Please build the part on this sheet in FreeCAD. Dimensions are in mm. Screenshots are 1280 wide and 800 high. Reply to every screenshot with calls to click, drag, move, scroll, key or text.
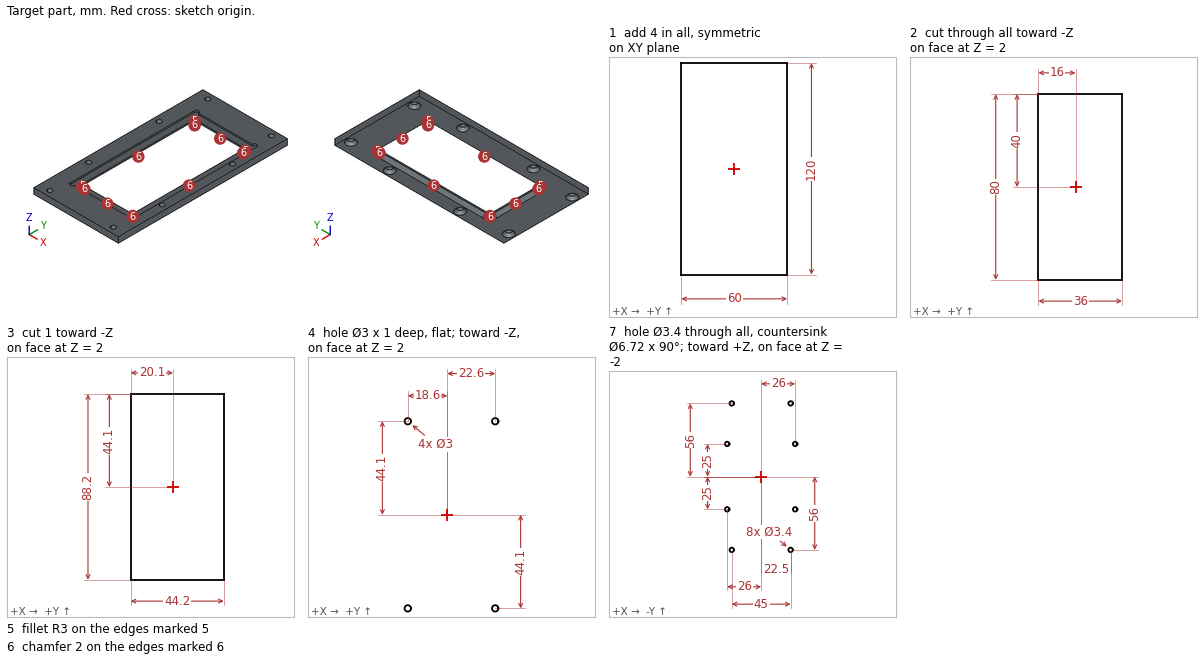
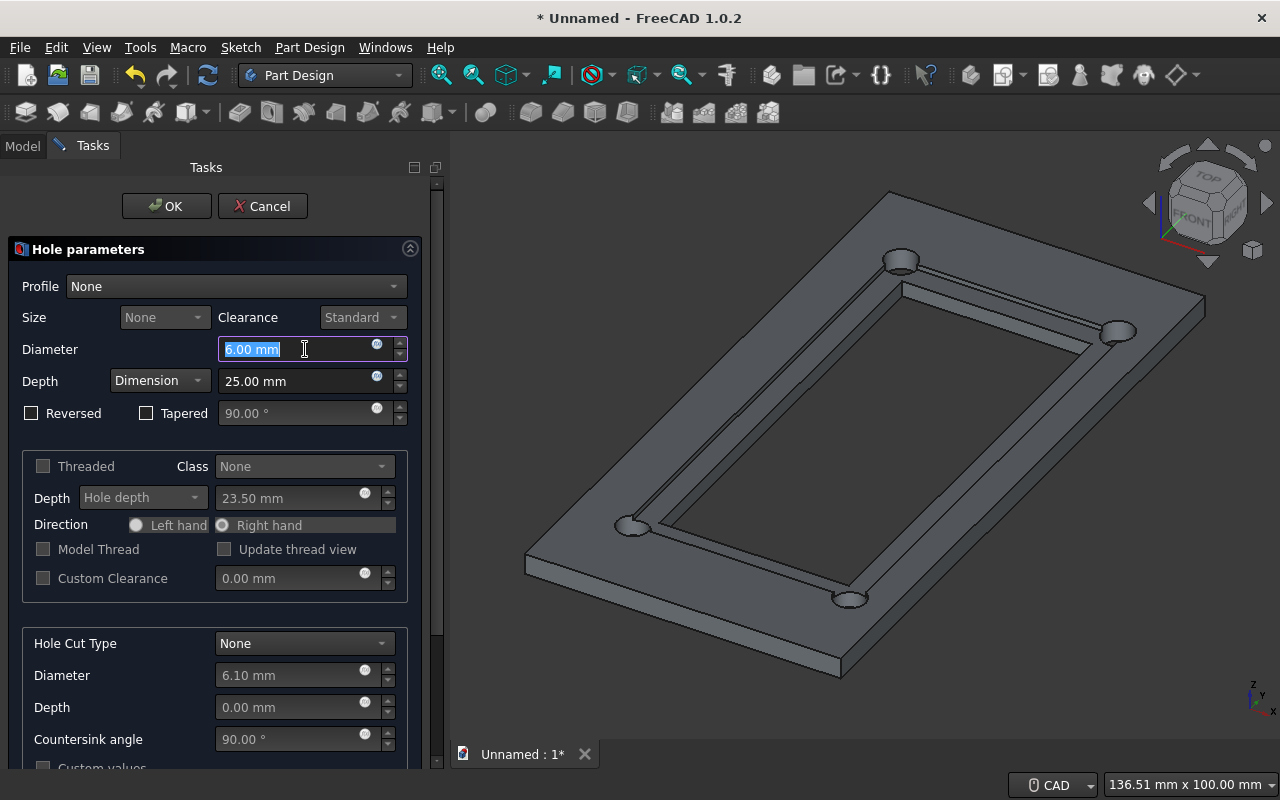
text(3)
key(Tab)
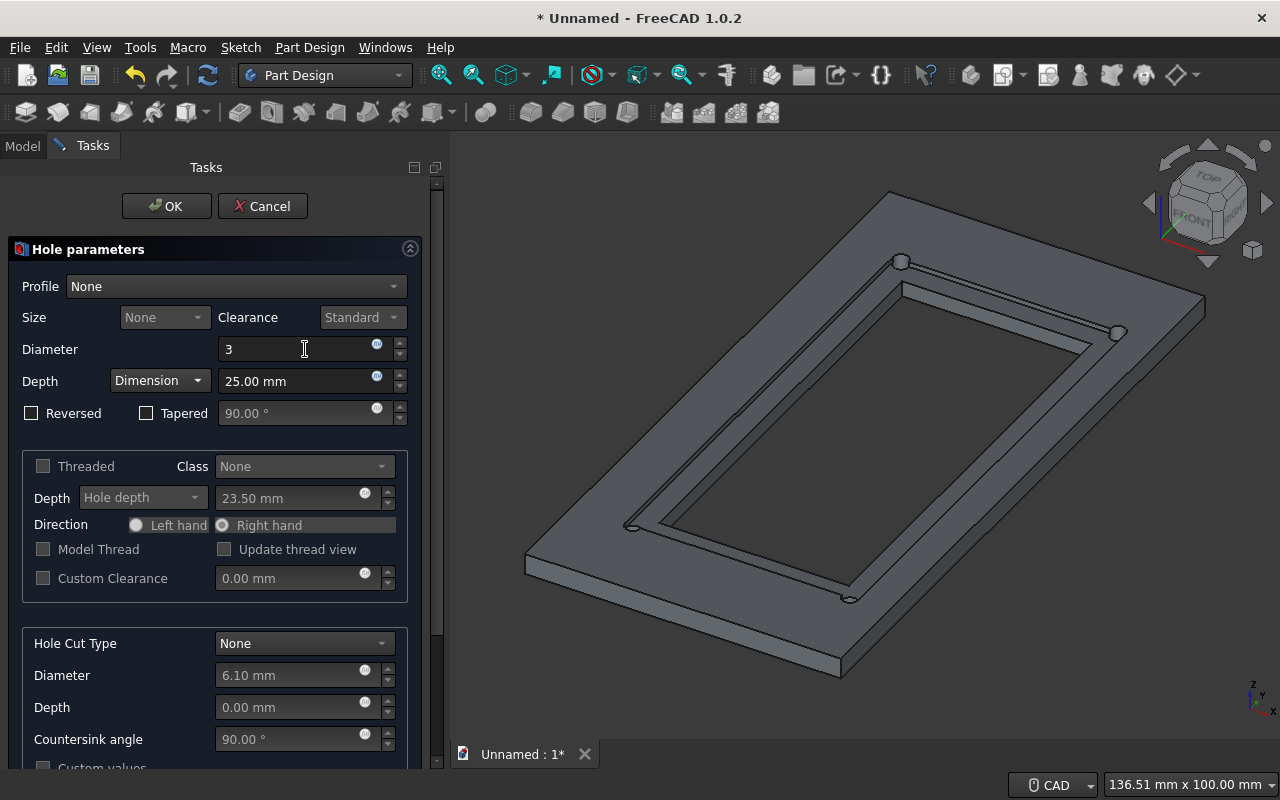
triple_click(305, 381)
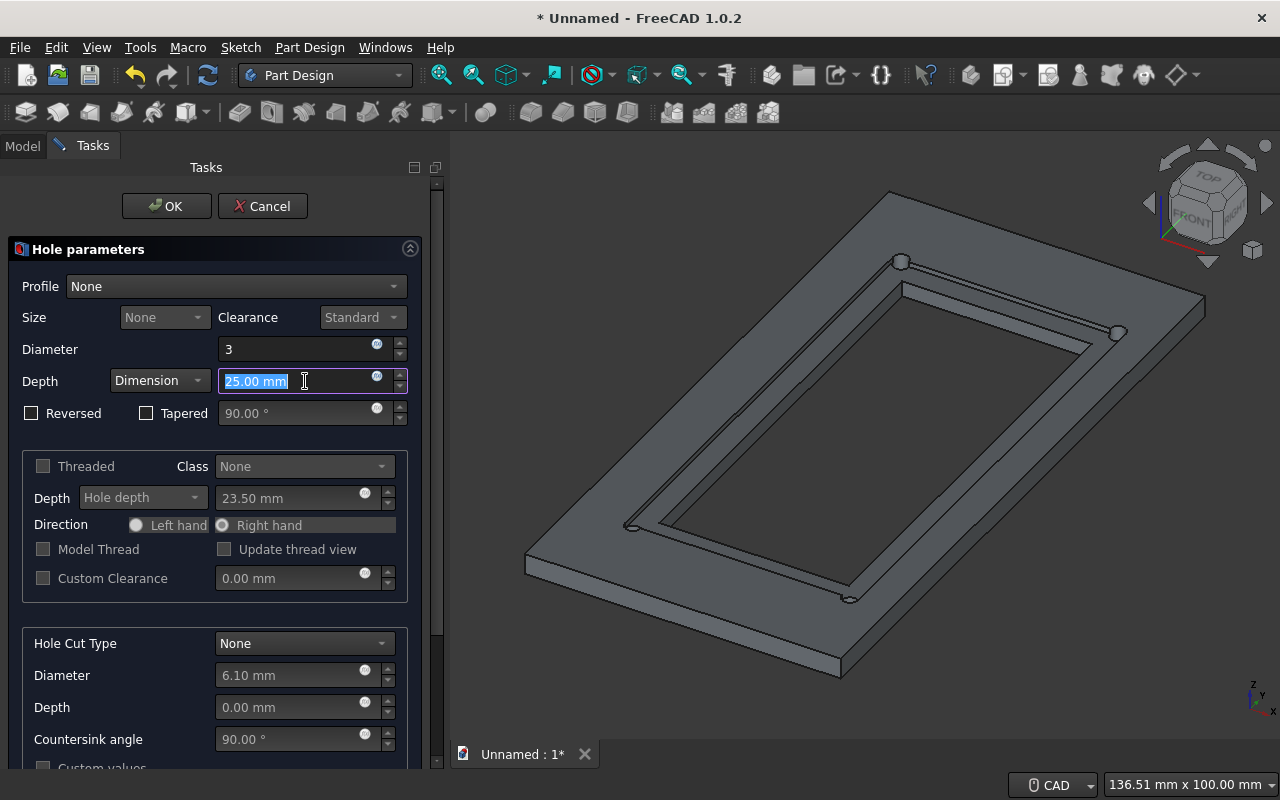
text(1)
key(Tab)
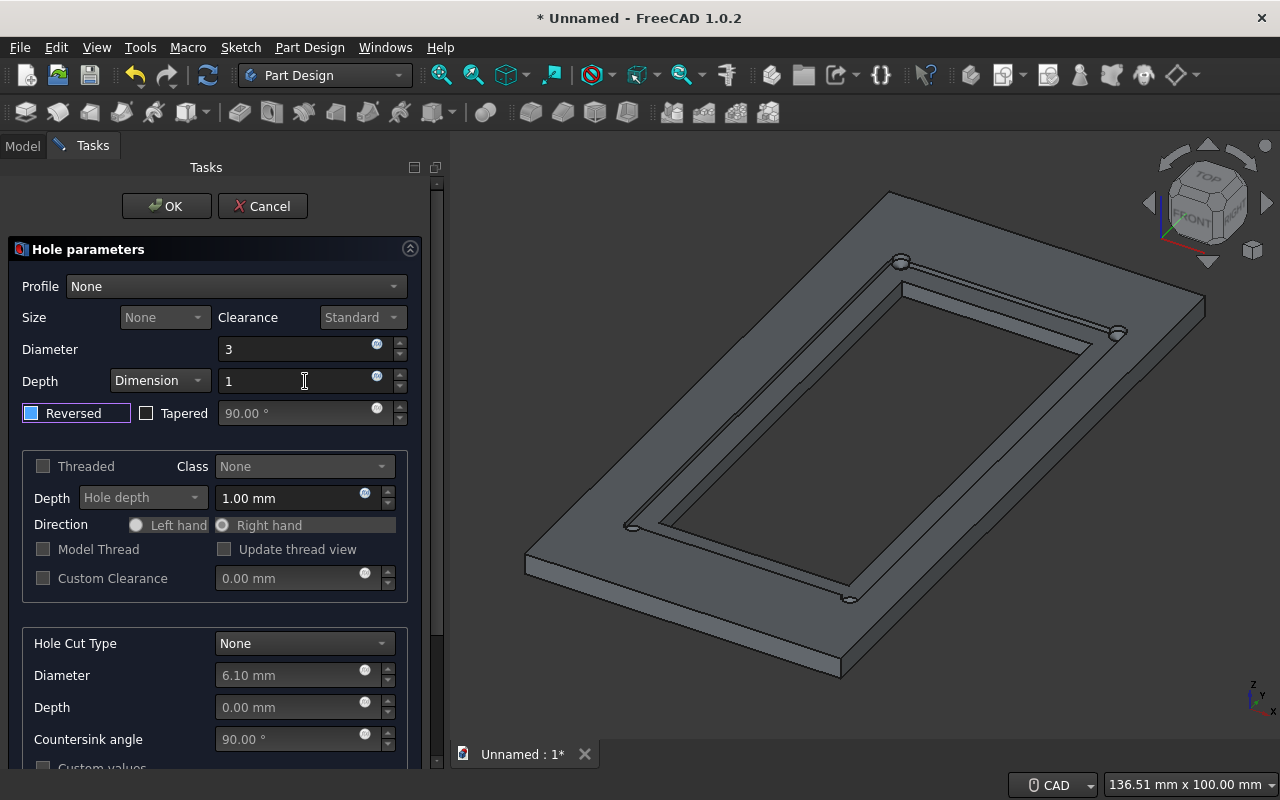
scroll(437, 472, down, 3)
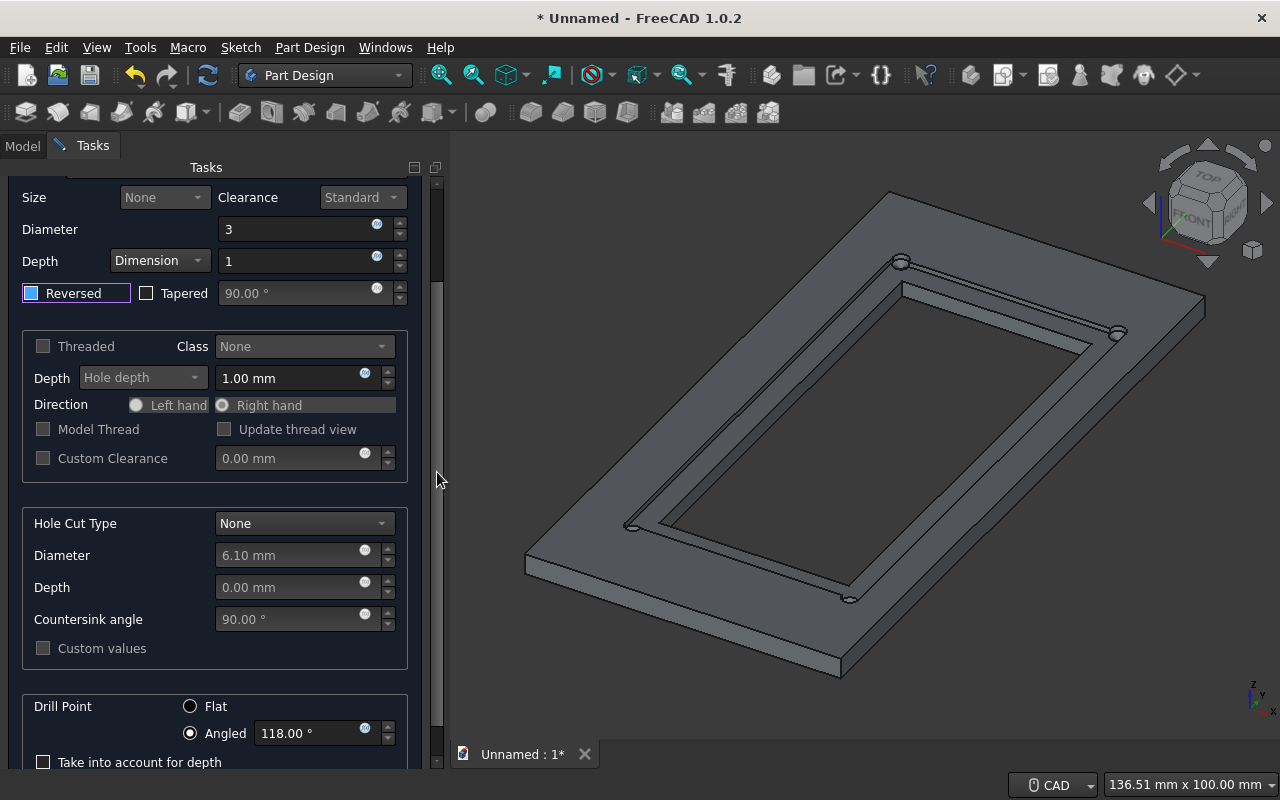
click(191, 669)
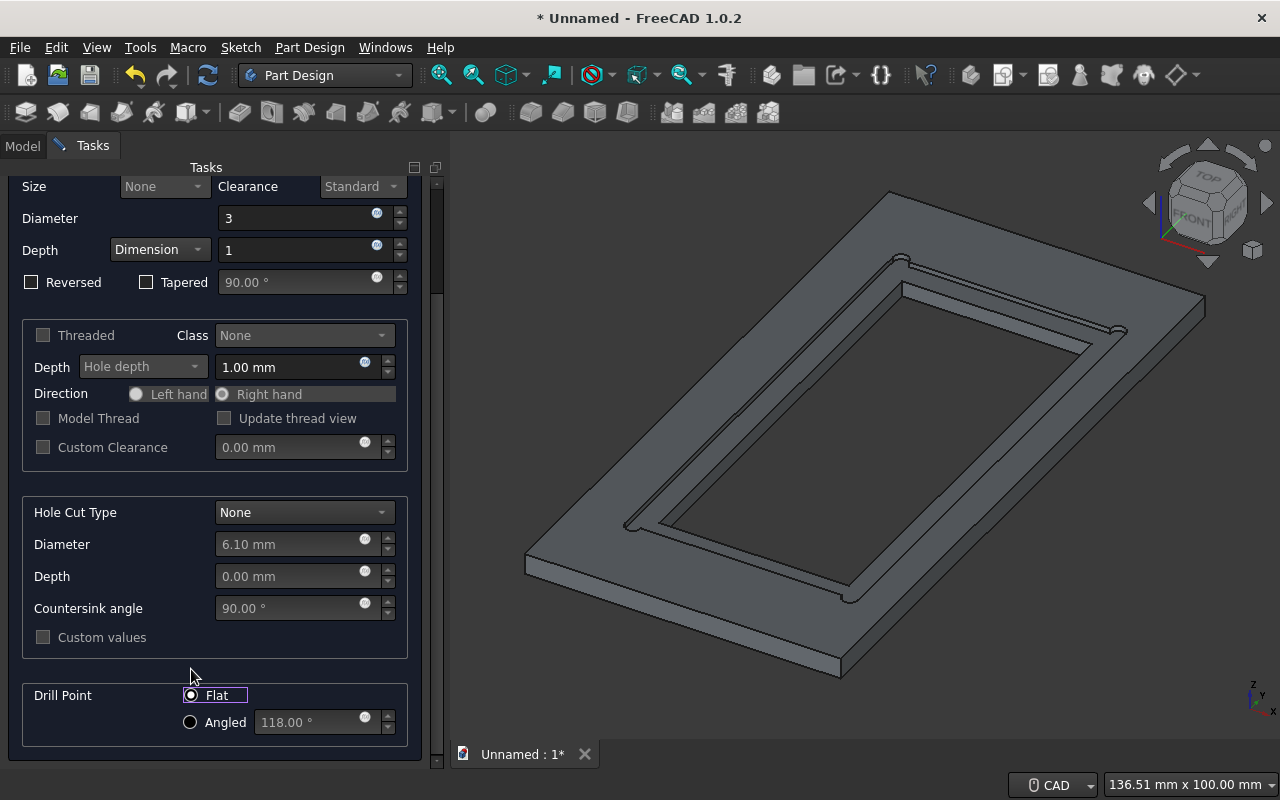
scroll(437, 472, up, 3)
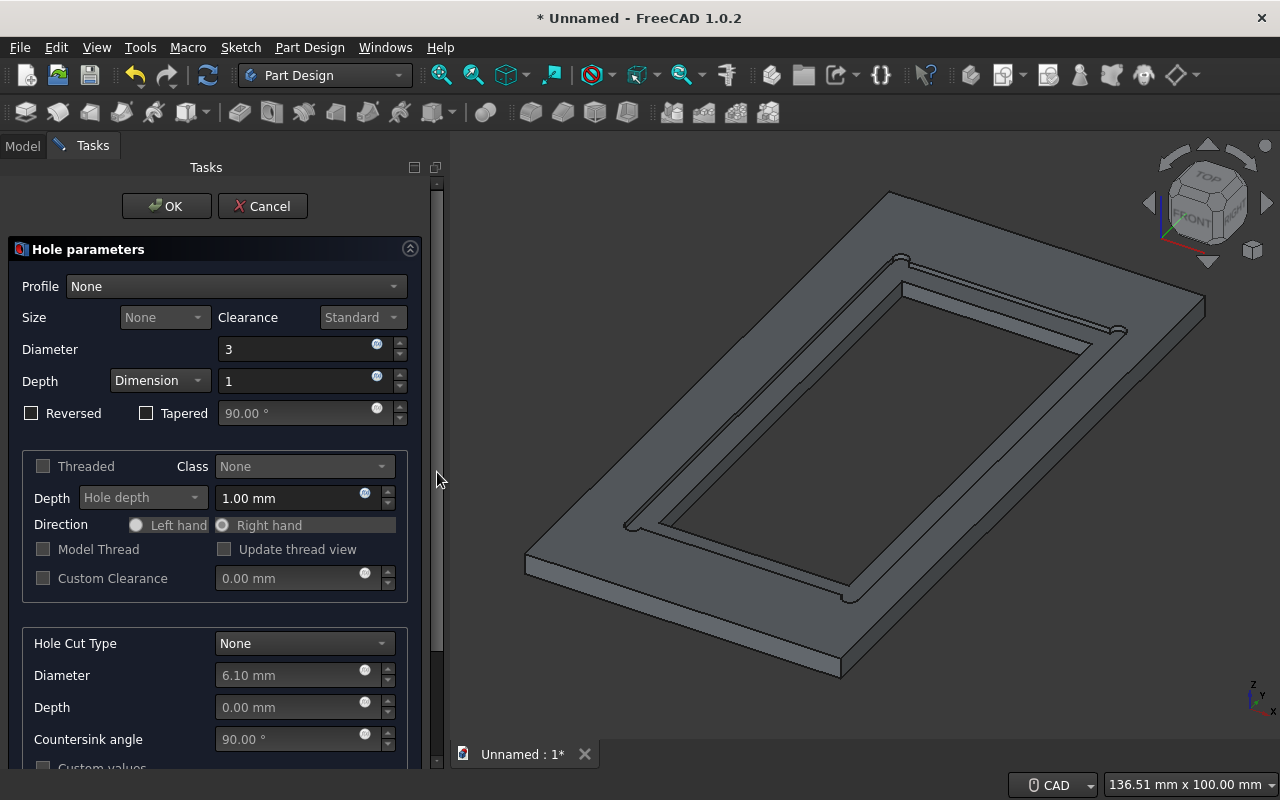
click(167, 206)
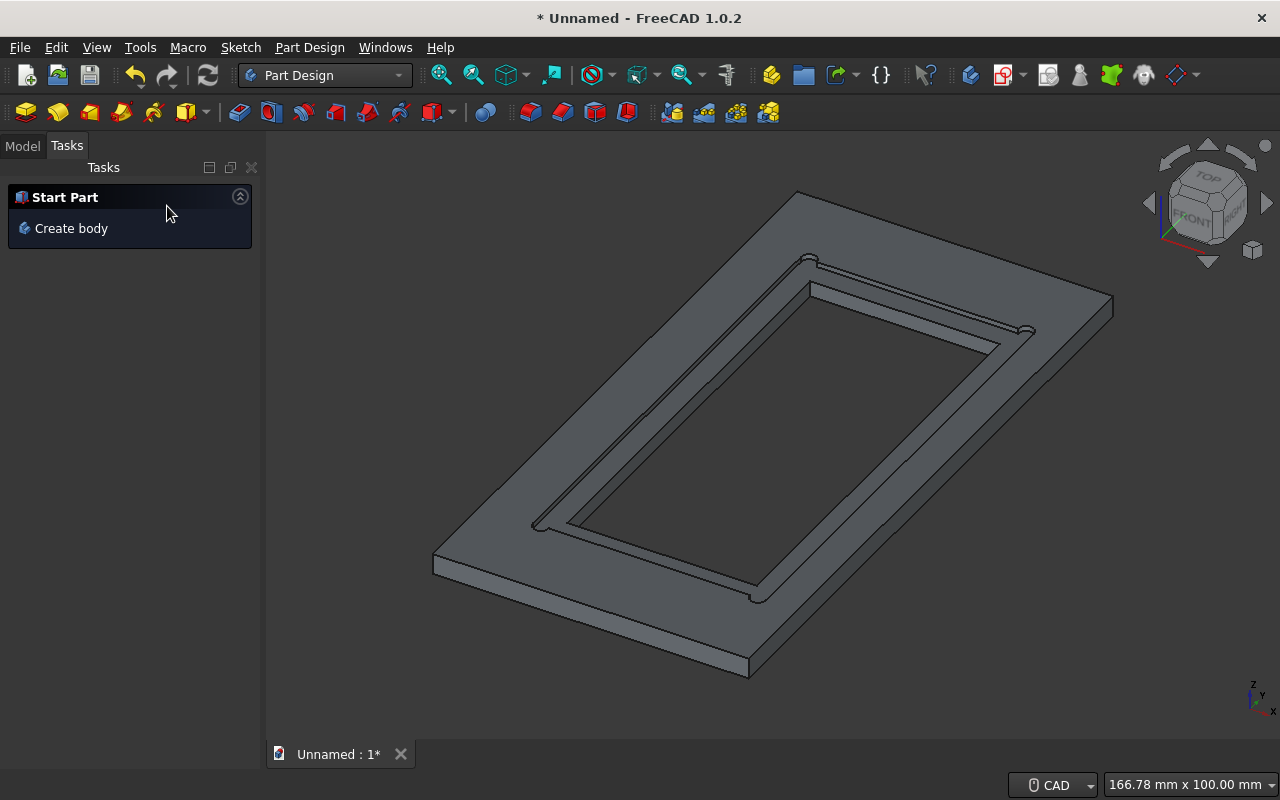
scroll(567, 529, up, 4)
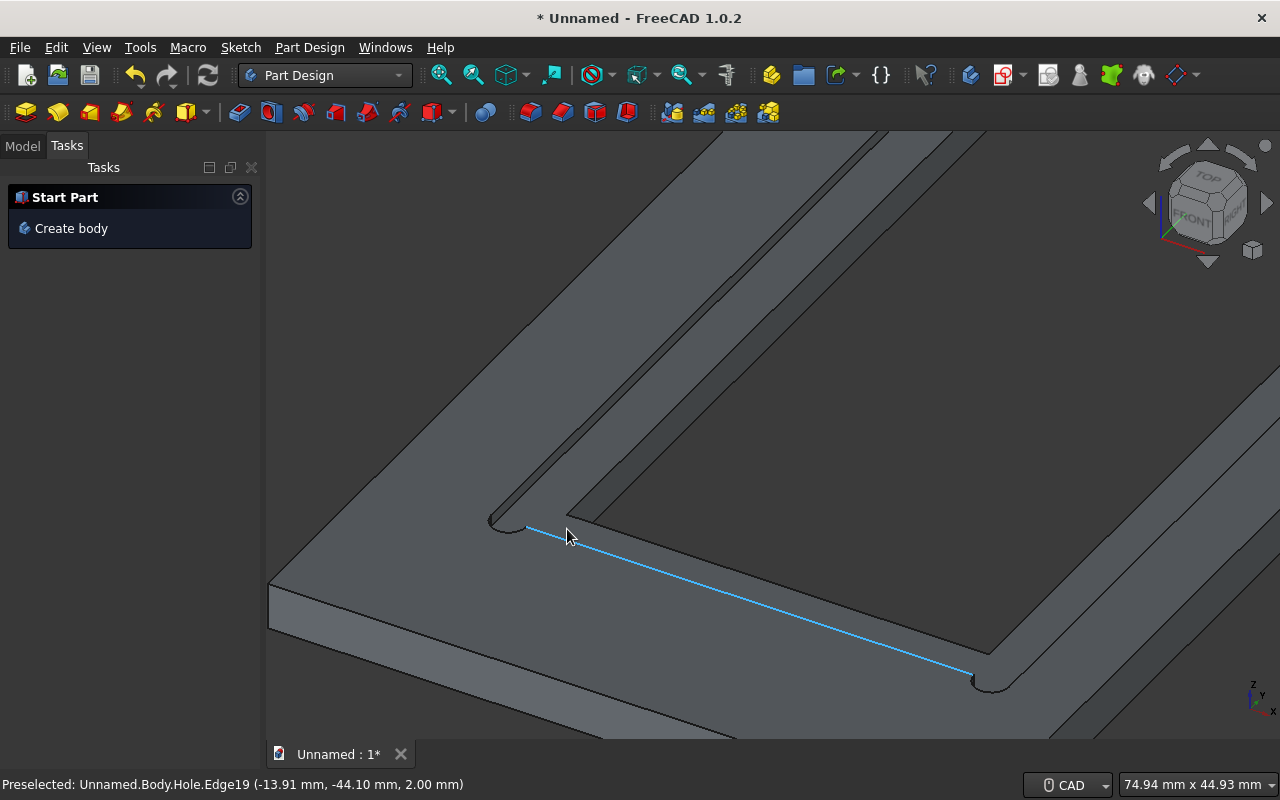
click(442, 76)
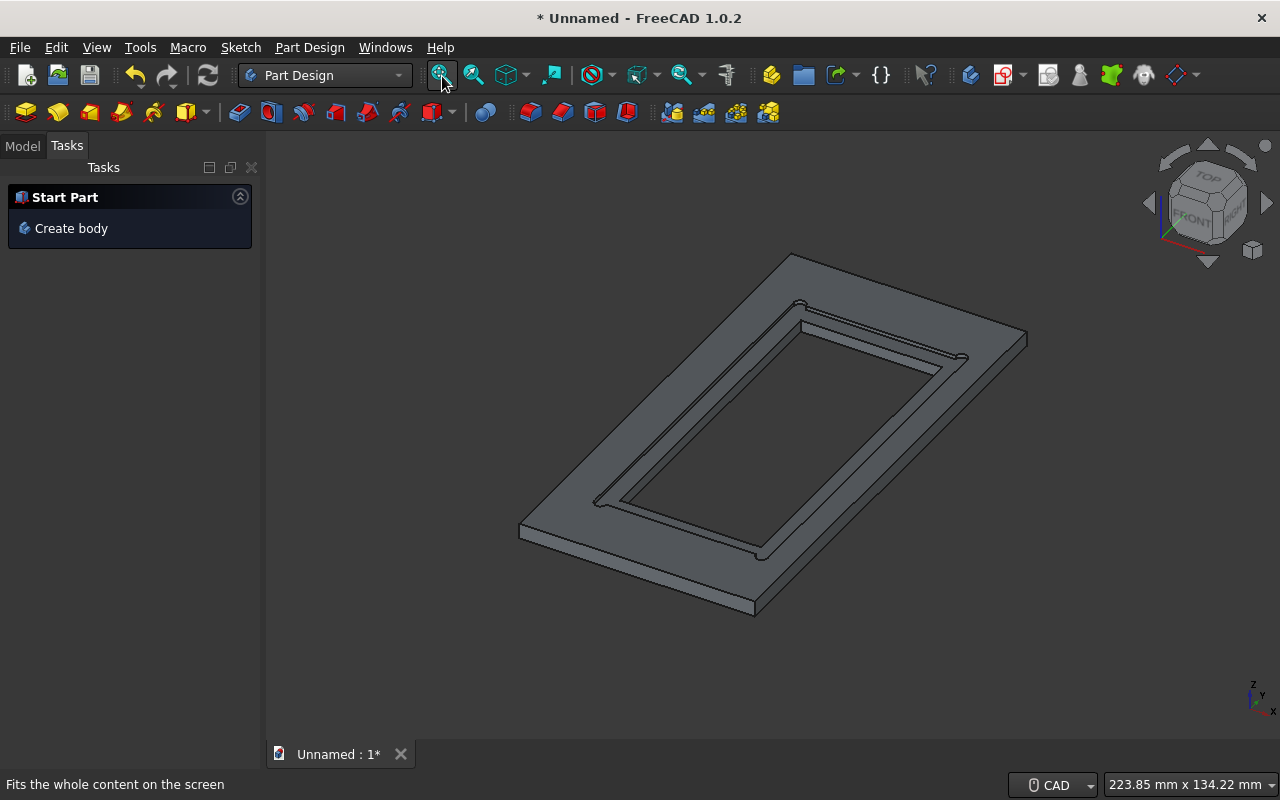
key(0)